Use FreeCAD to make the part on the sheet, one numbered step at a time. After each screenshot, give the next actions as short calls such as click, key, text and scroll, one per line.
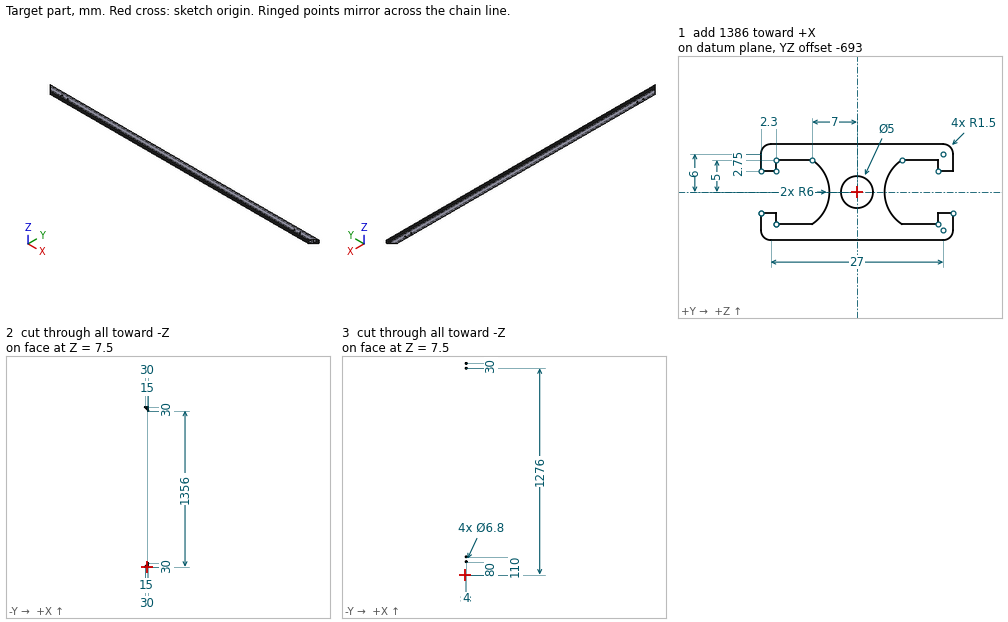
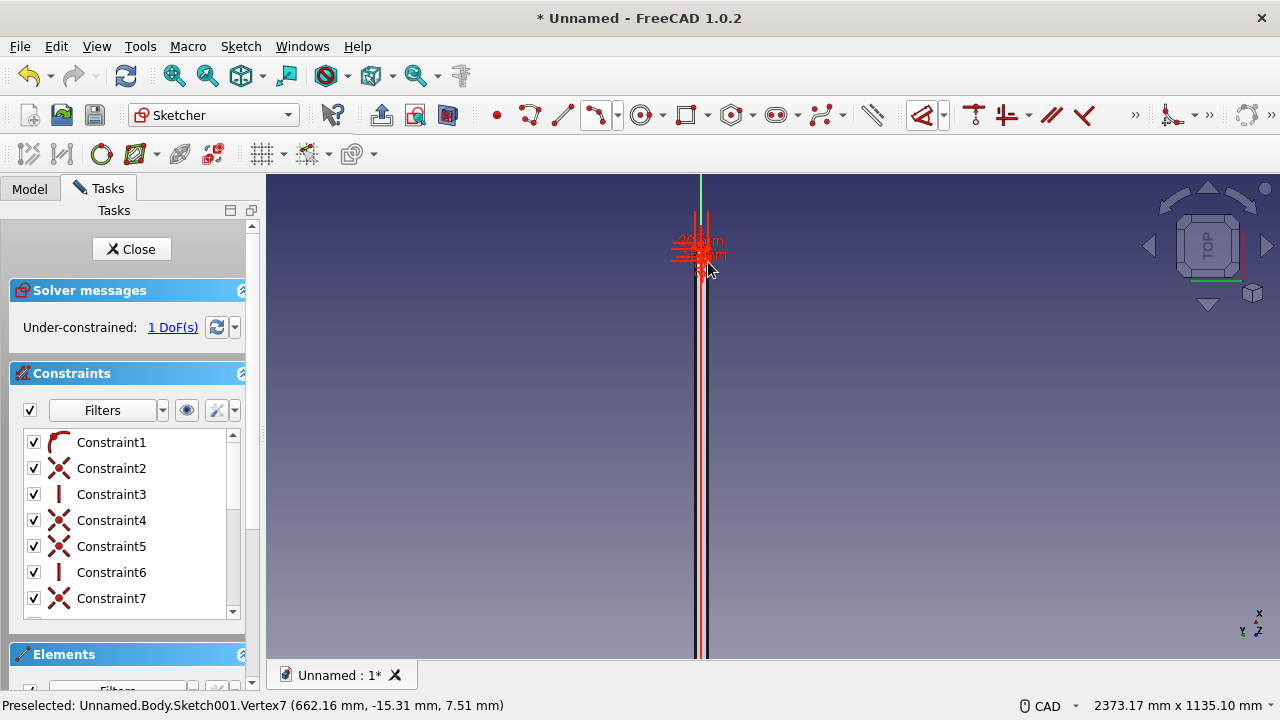
click(708, 261)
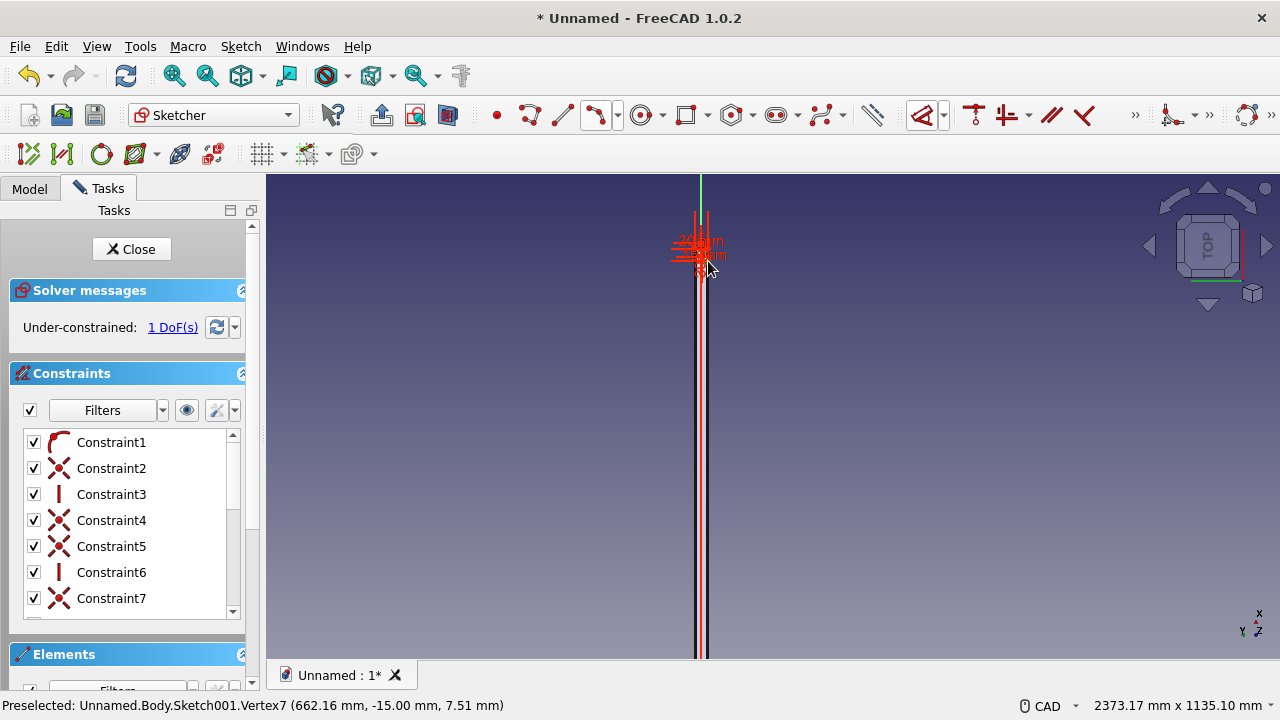
click(944, 116)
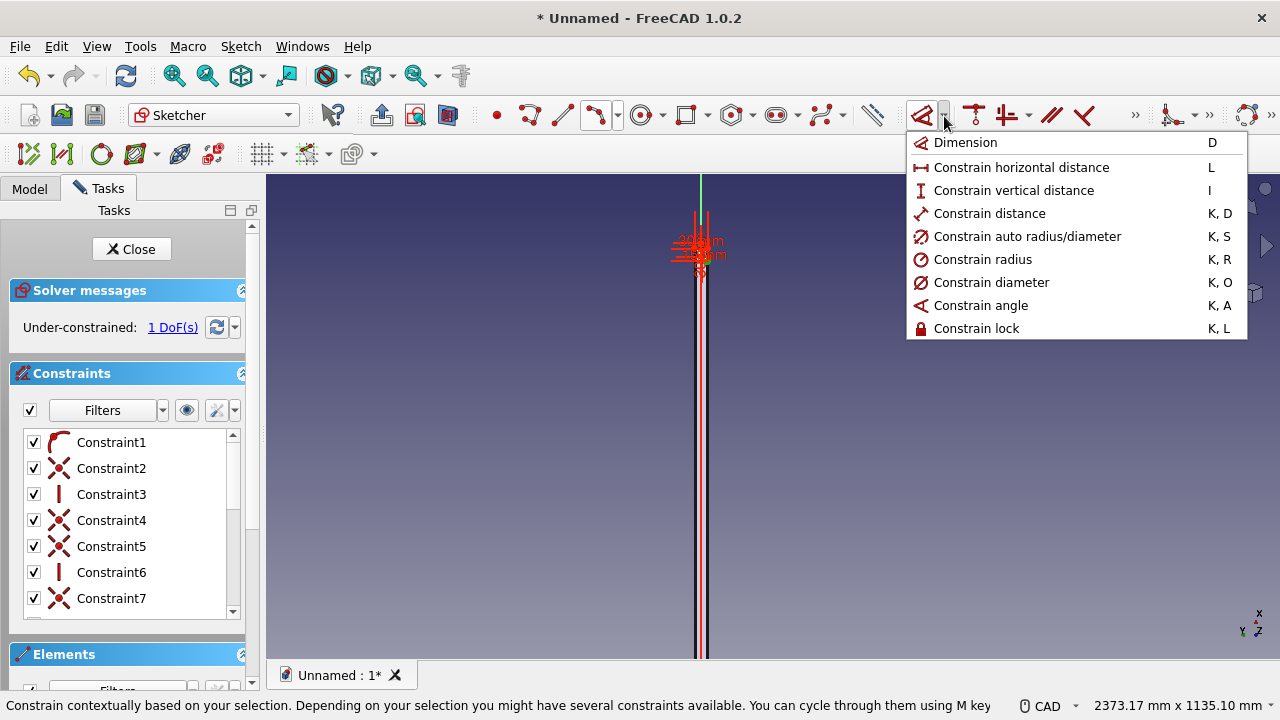
click(1077, 190)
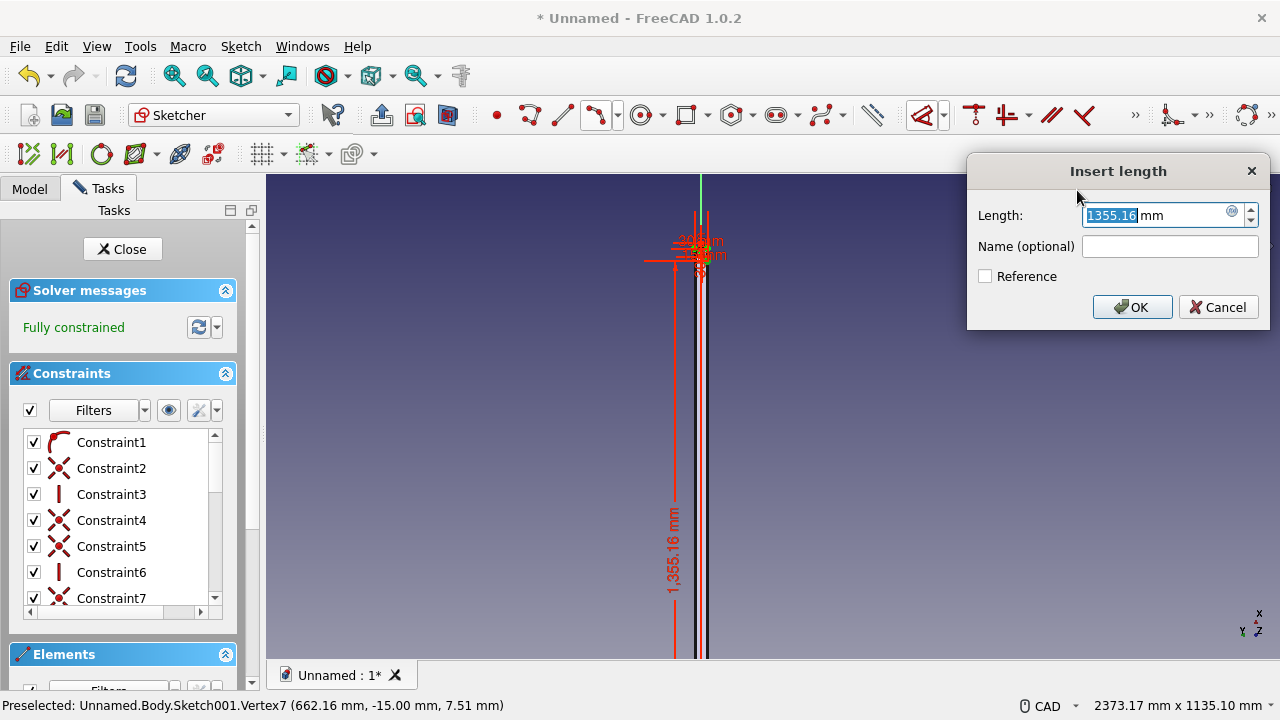
text(1356)
key(Return)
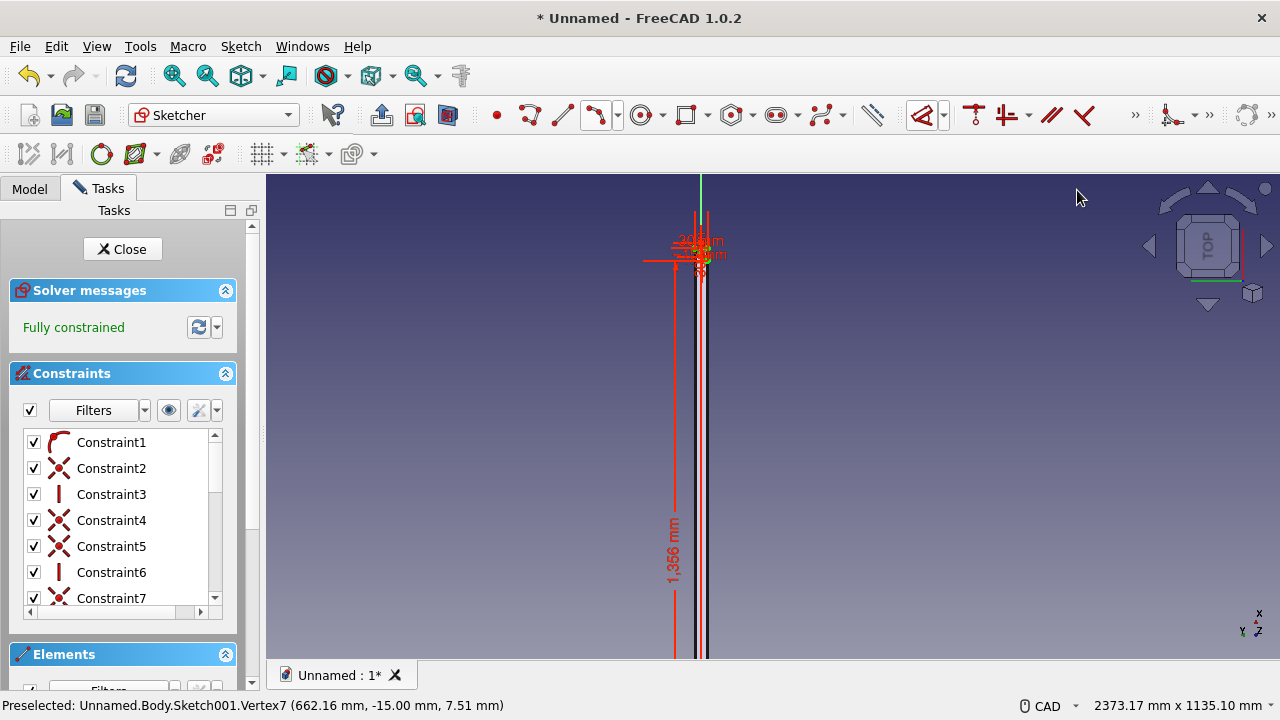
click(123, 249)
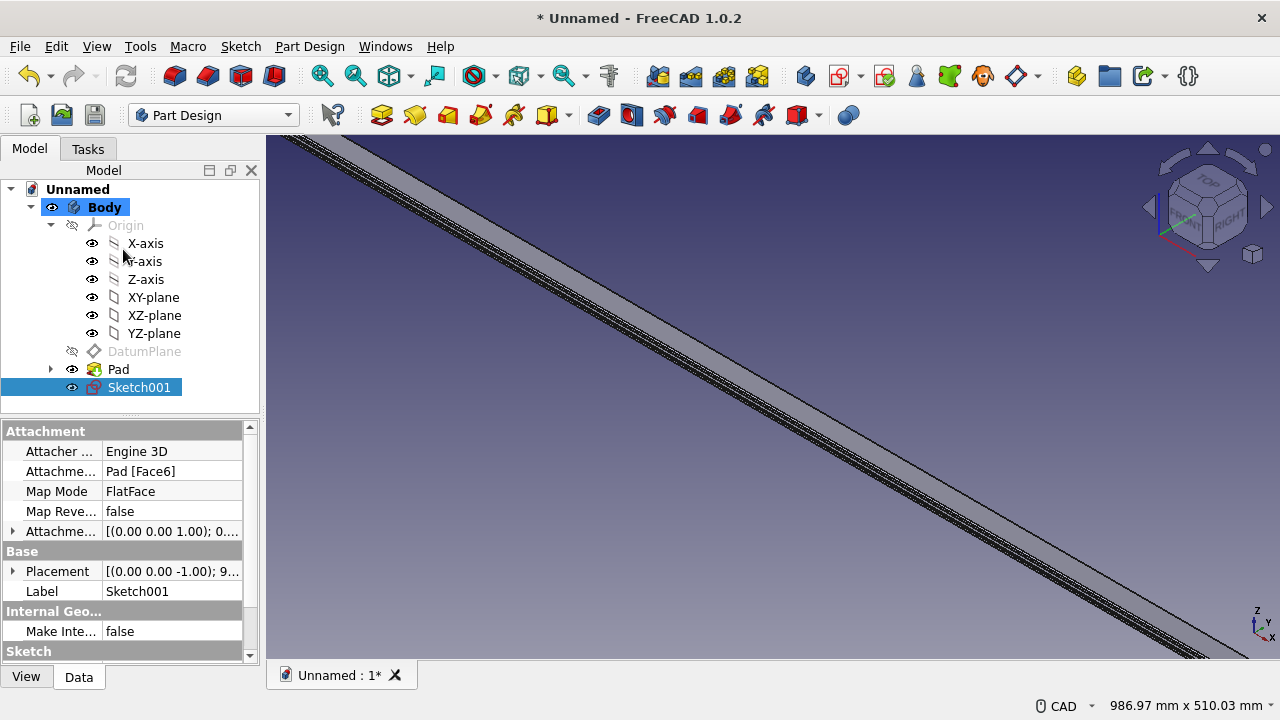
click(599, 116)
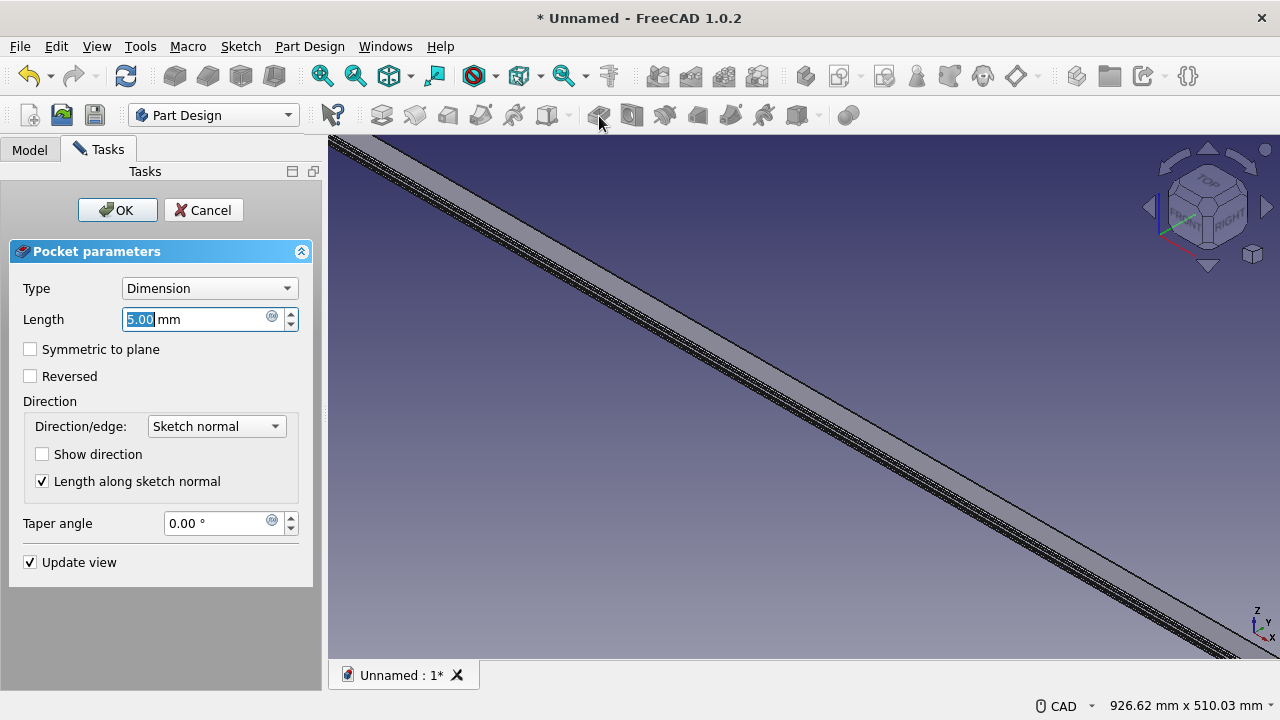
click(210, 288)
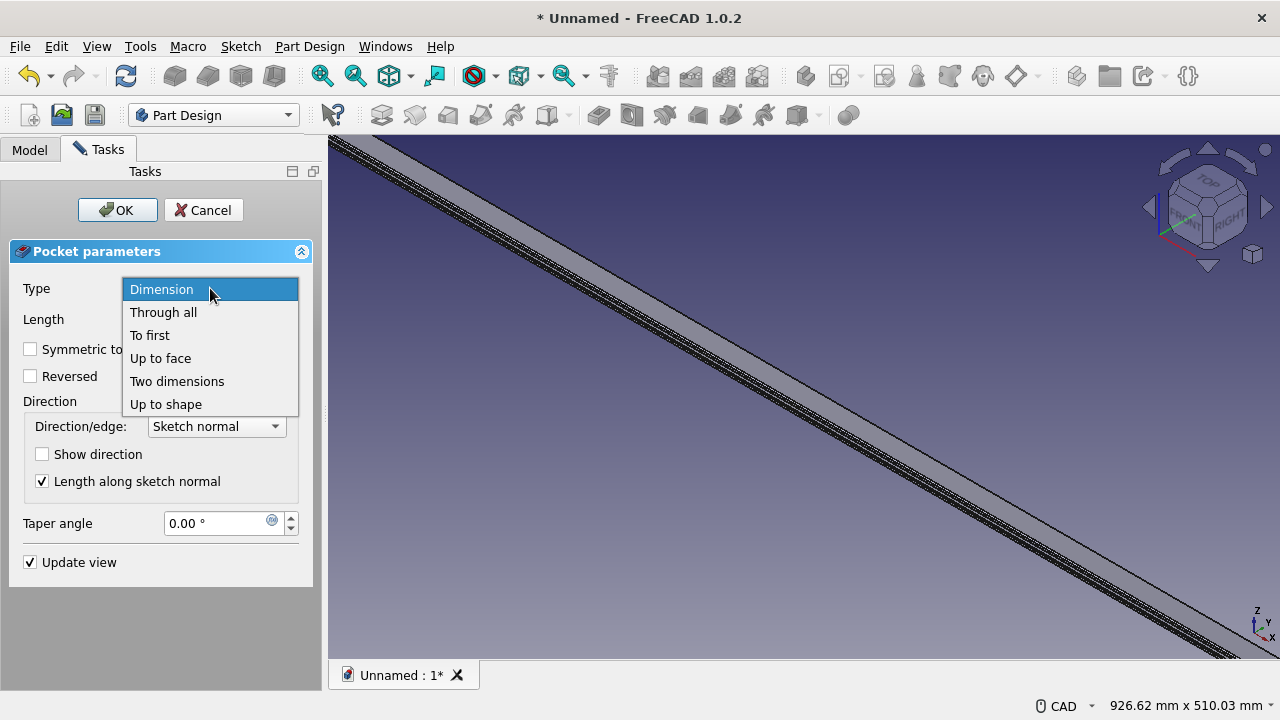
click(208, 312)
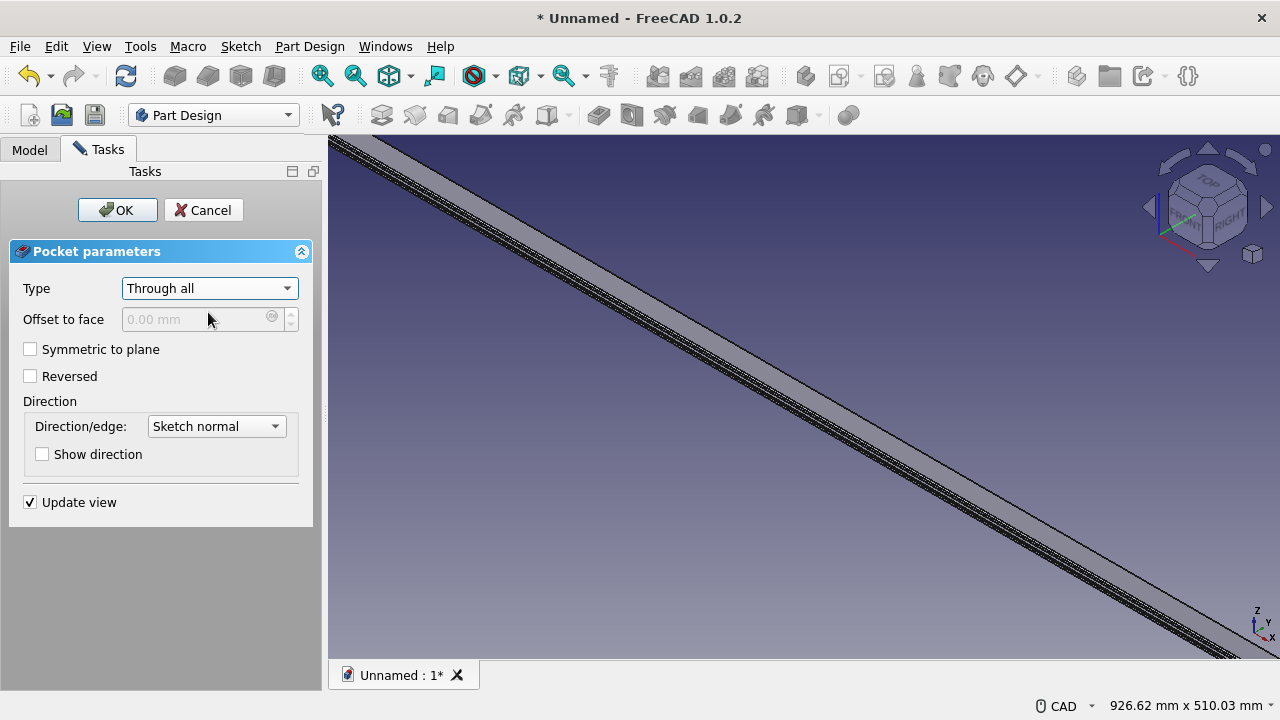
click(118, 210)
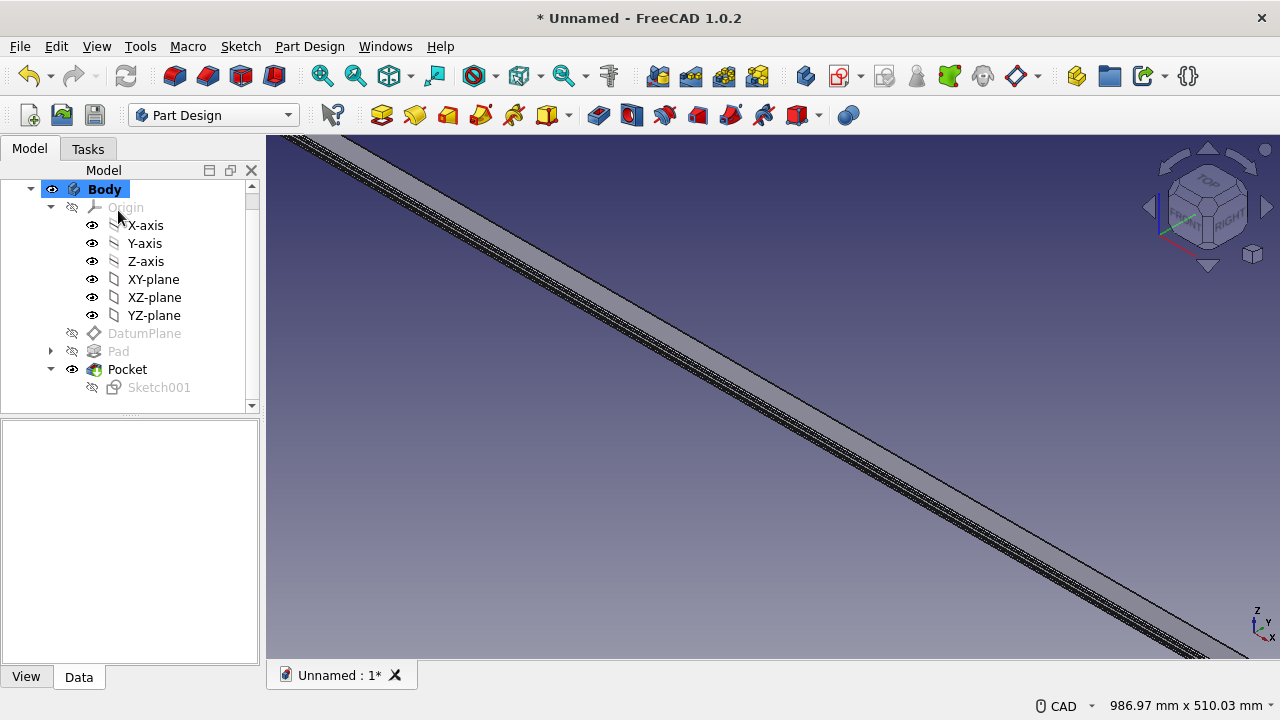
click(323, 76)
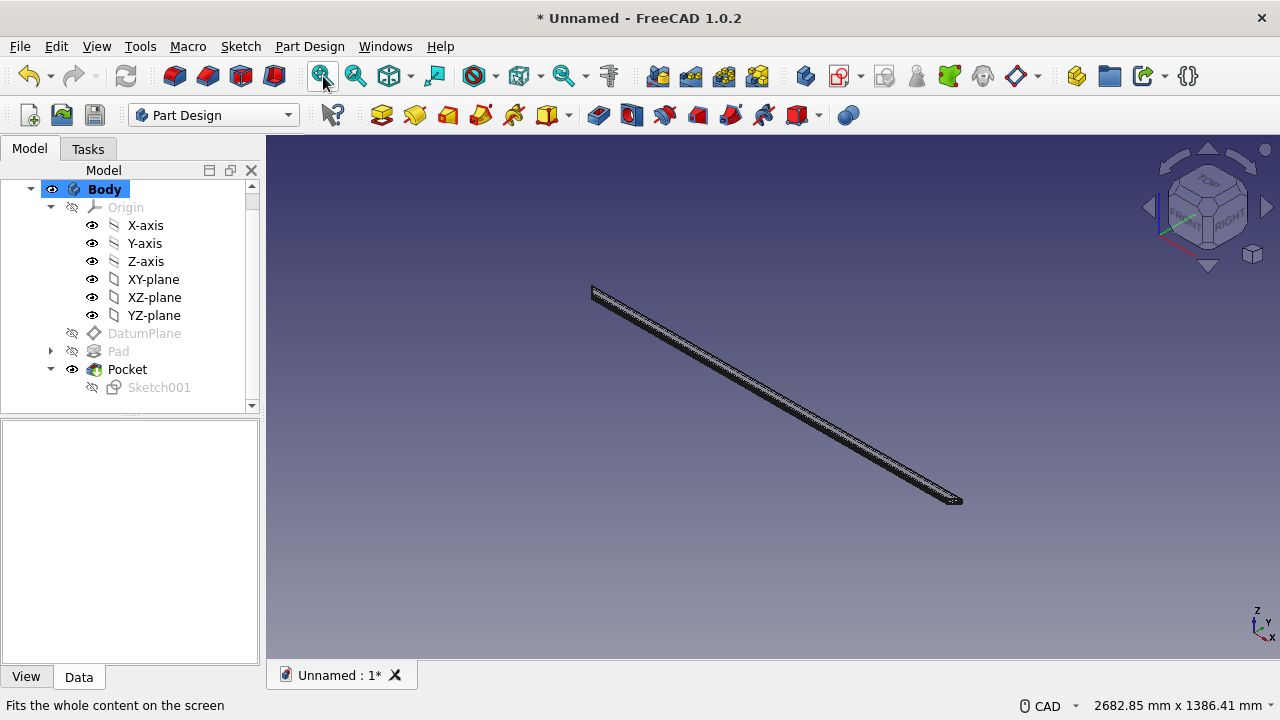
scroll(826, 424, up, 5)